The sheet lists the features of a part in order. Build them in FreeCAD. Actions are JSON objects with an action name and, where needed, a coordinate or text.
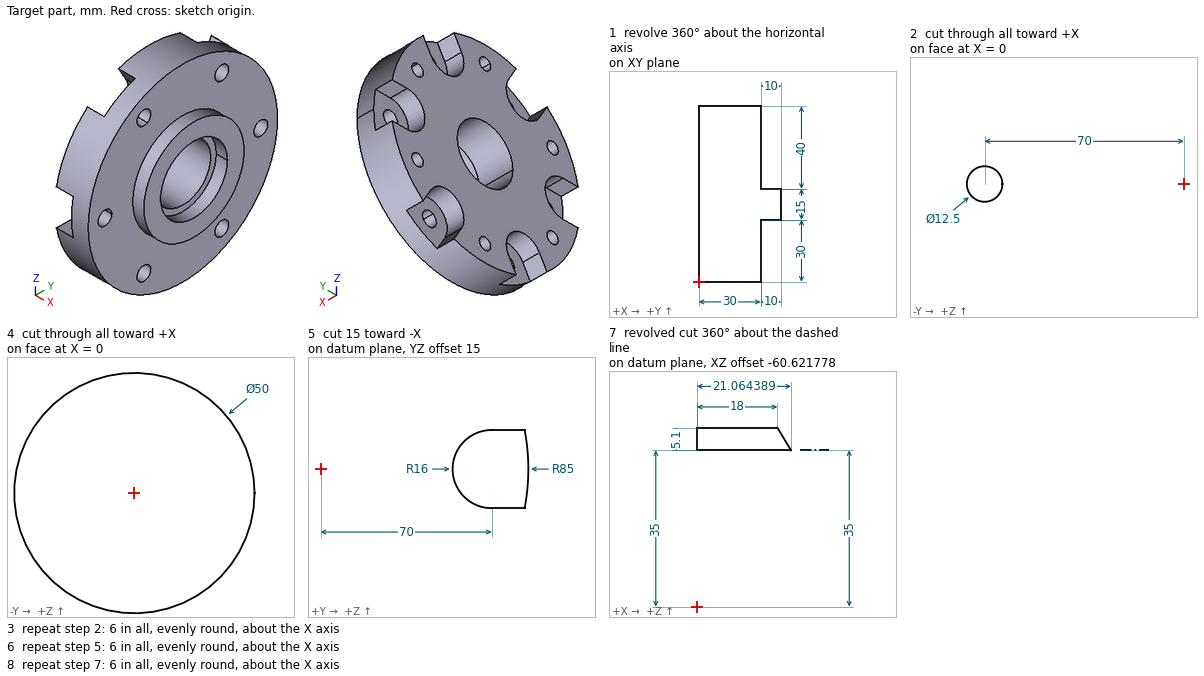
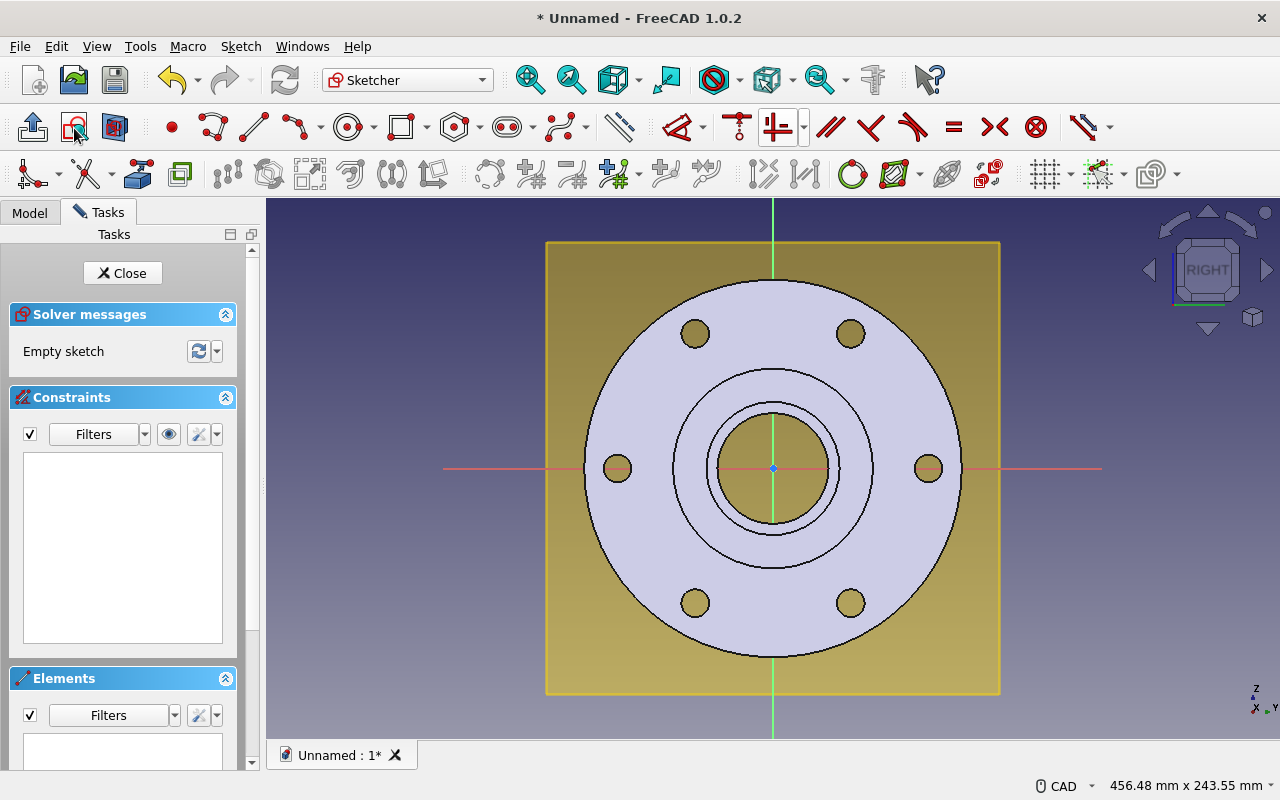
{"action": "left_click", "coordinate": [115, 128]}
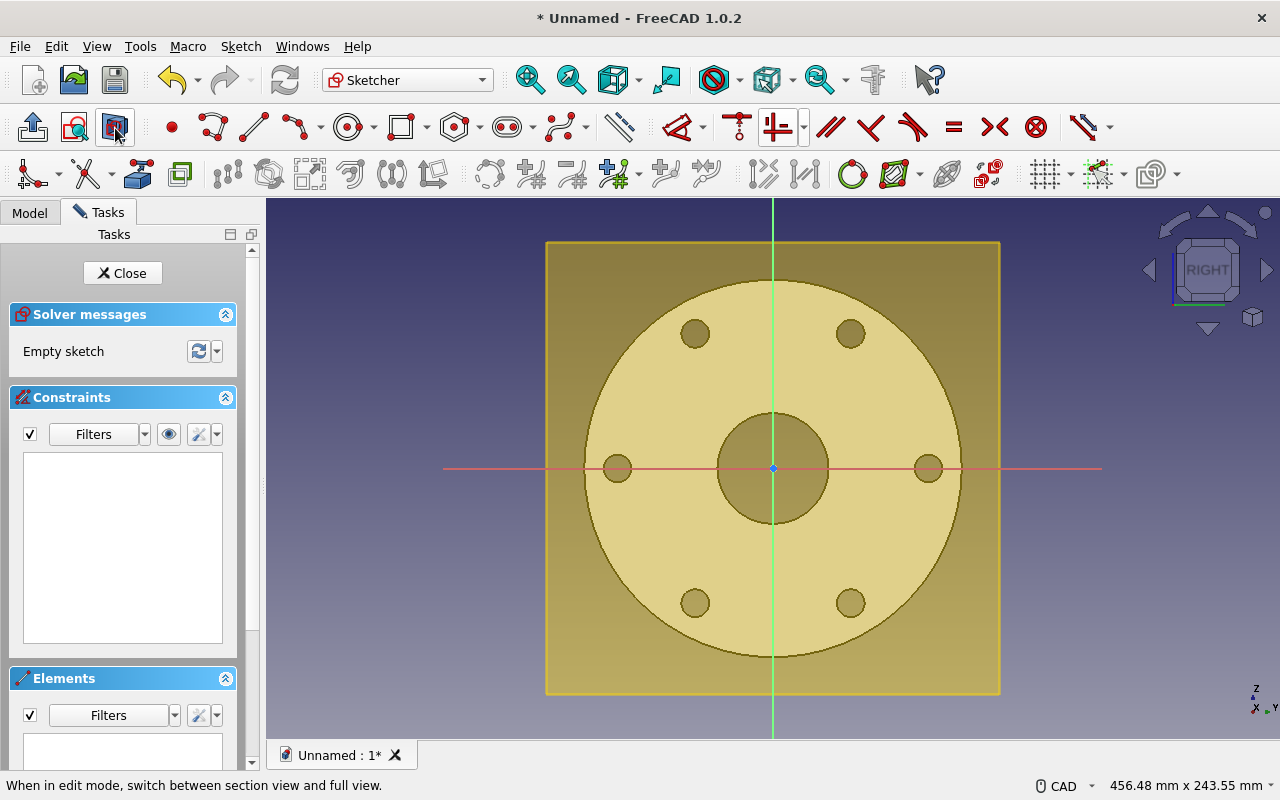
{"action": "scroll", "coordinate": [984, 469], "scroll_direction": "up", "scroll_amount": 8}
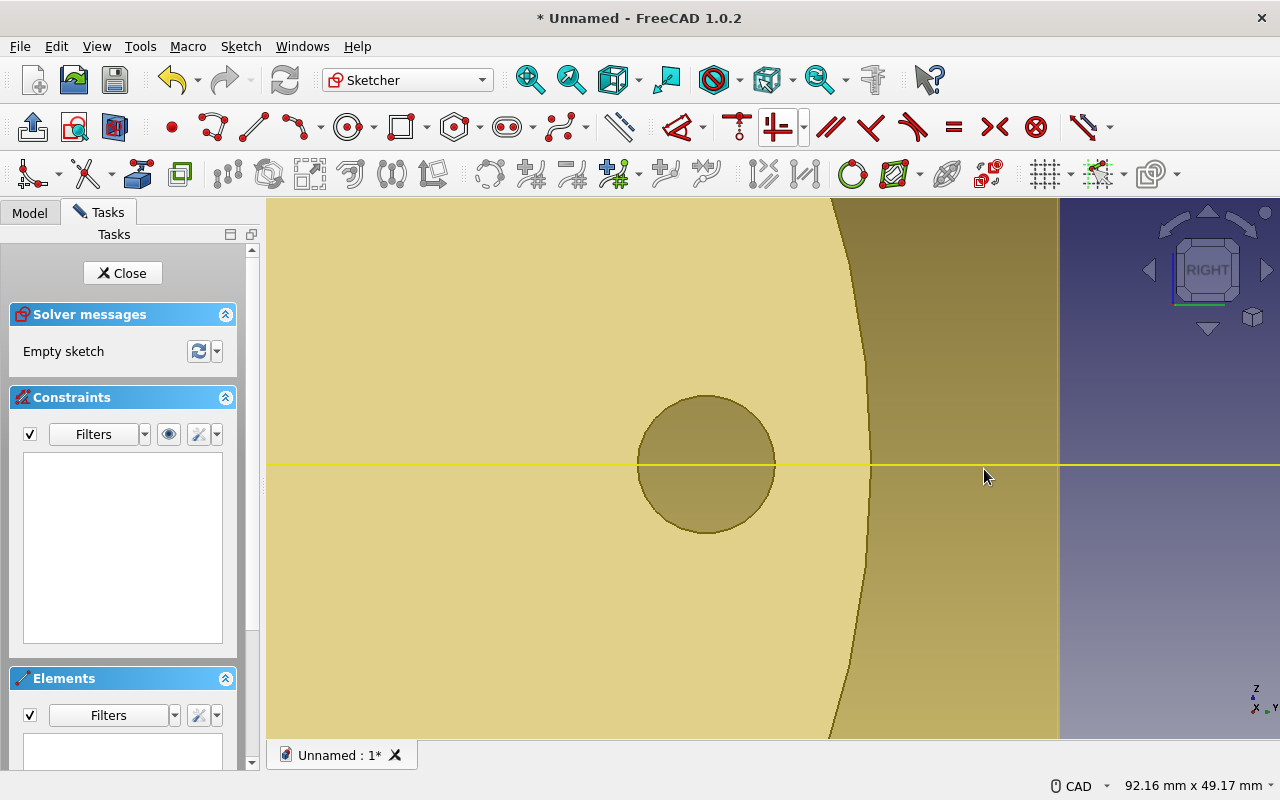
{"action": "left_click", "coordinate": [254, 128]}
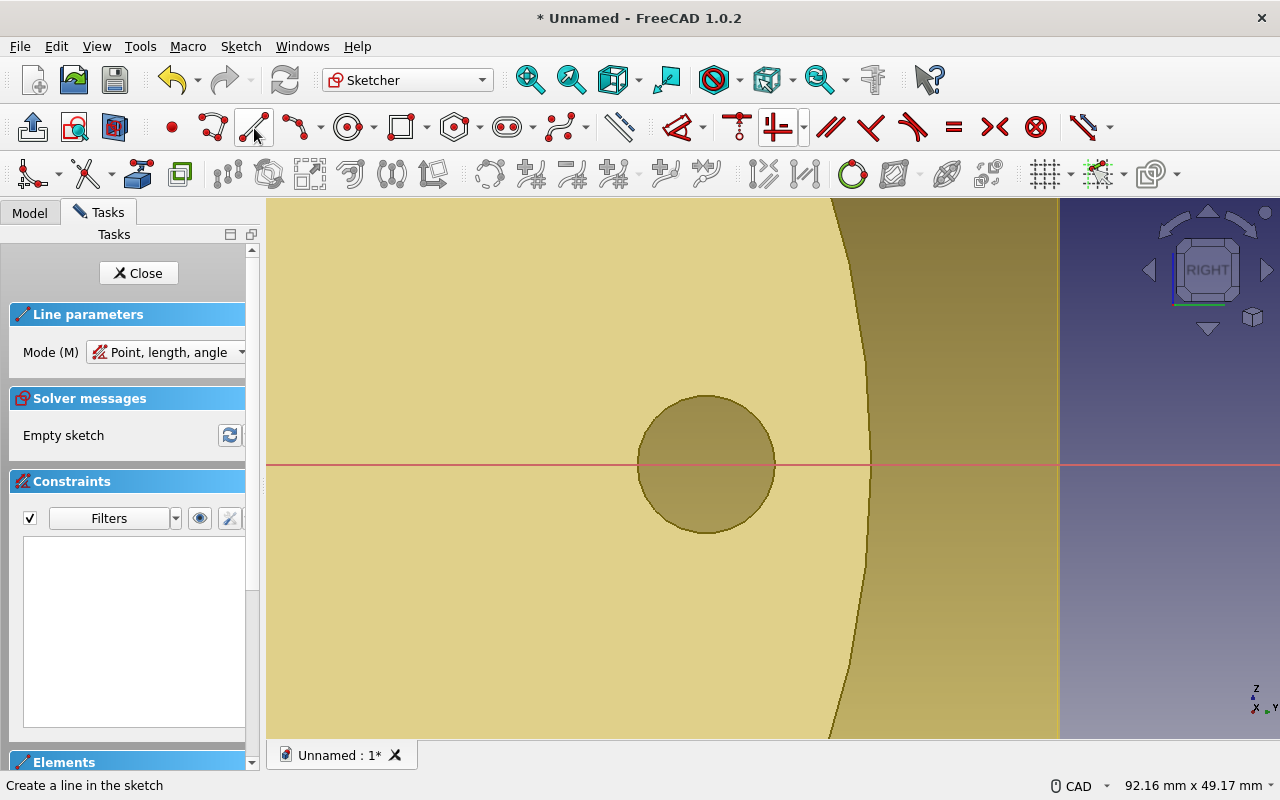
{"action": "left_click", "coordinate": [855, 641]}
{"action": "left_click", "coordinate": [706, 641]}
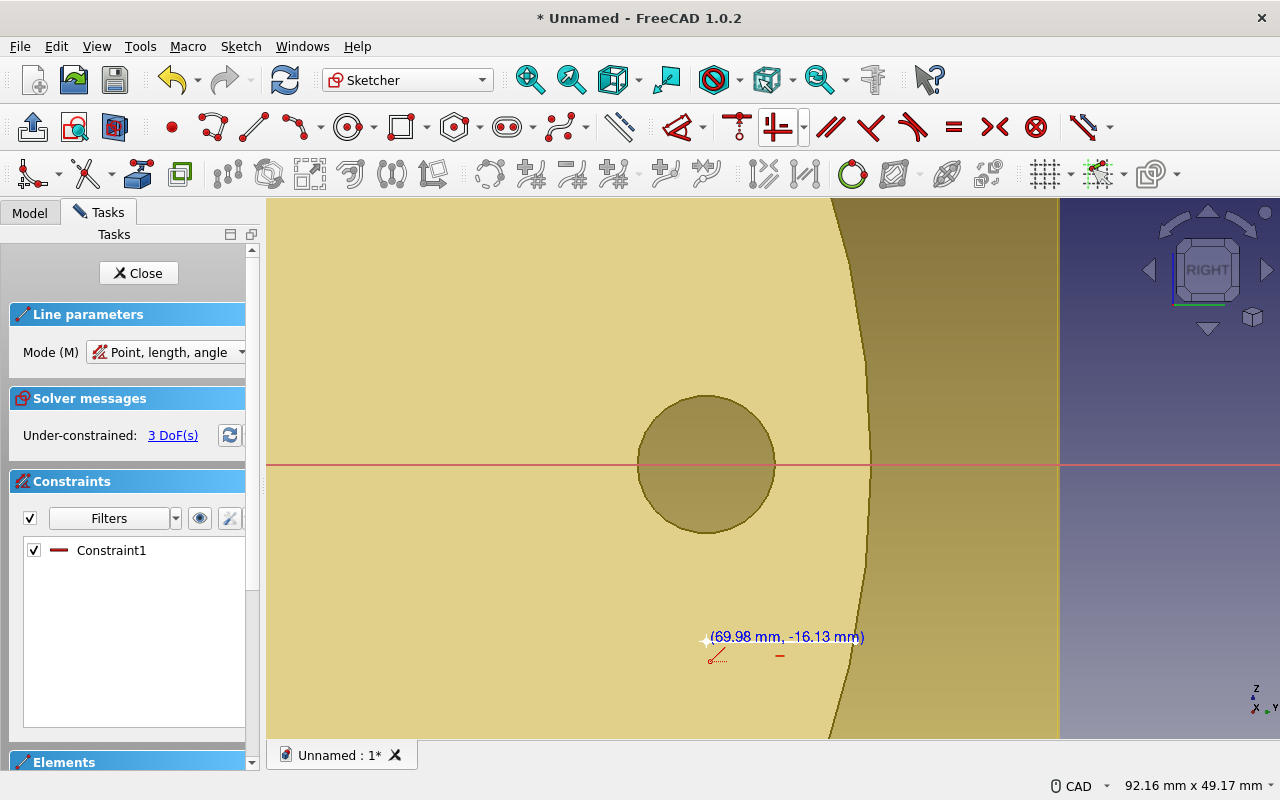
{"action": "left_click", "coordinate": [706, 289]}
{"action": "left_click", "coordinate": [855, 289]}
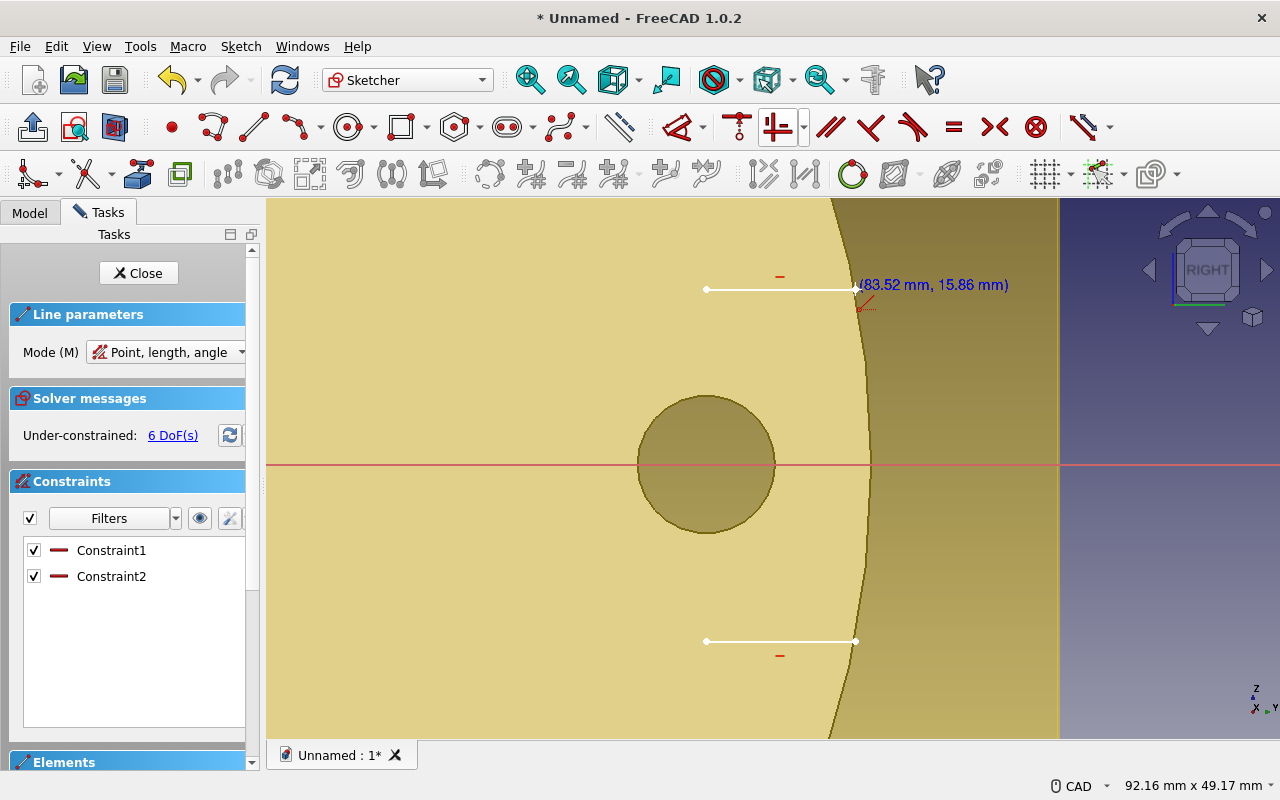
{"action": "left_click", "coordinate": [294, 128]}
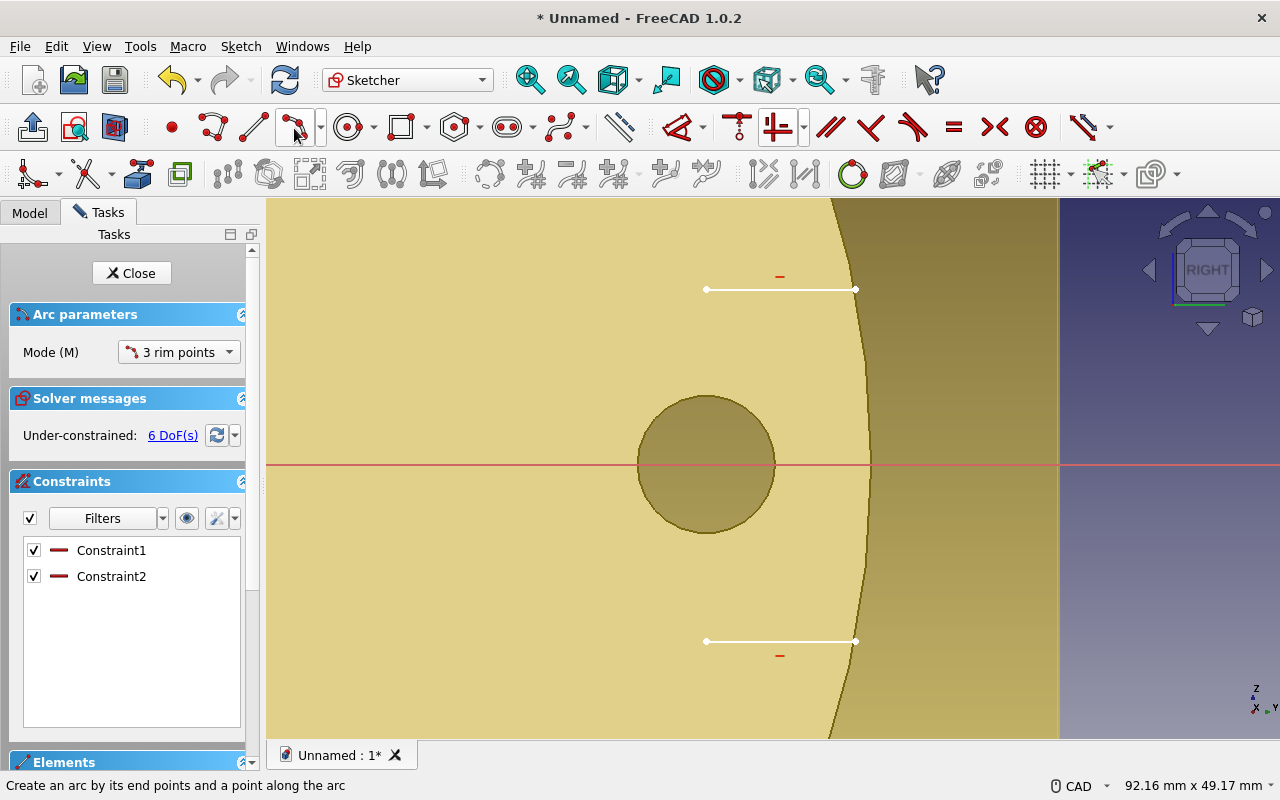
{"action": "left_click", "coordinate": [706, 642]}
{"action": "left_click", "coordinate": [706, 290]}
{"action": "left_click", "coordinate": [539, 410]}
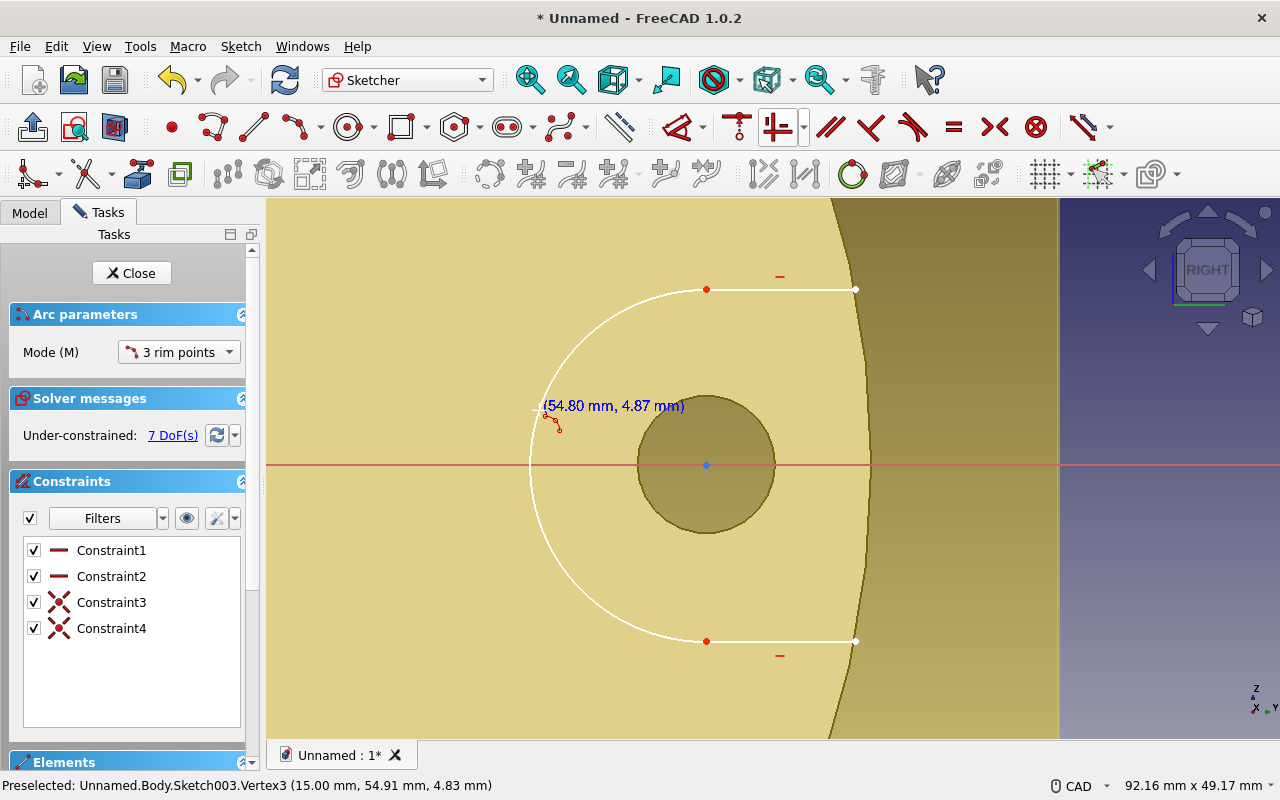
{"action": "left_click", "coordinate": [855, 290]}
{"action": "left_click", "coordinate": [855, 642]}
{"action": "left_click", "coordinate": [871, 500]}
{"action": "key", "text": "Escape"}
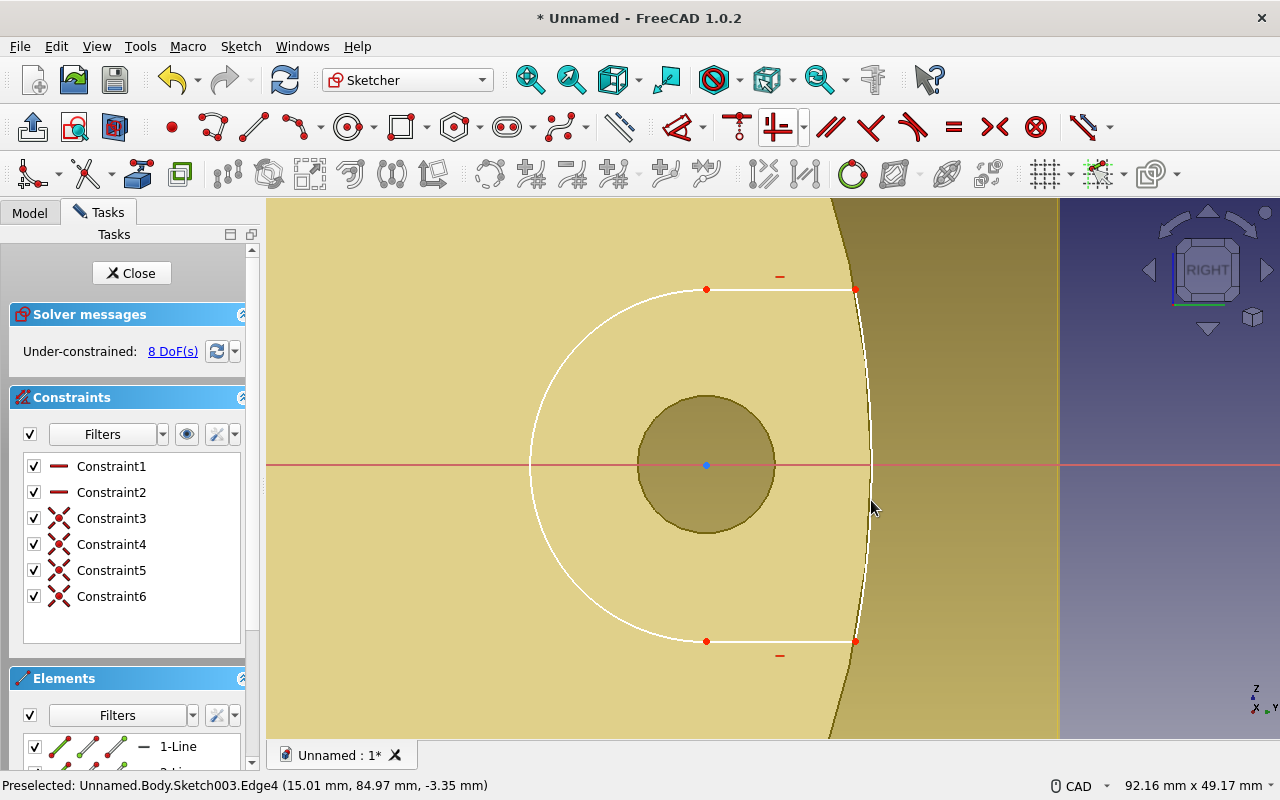
{"action": "left_click", "coordinate": [810, 642]}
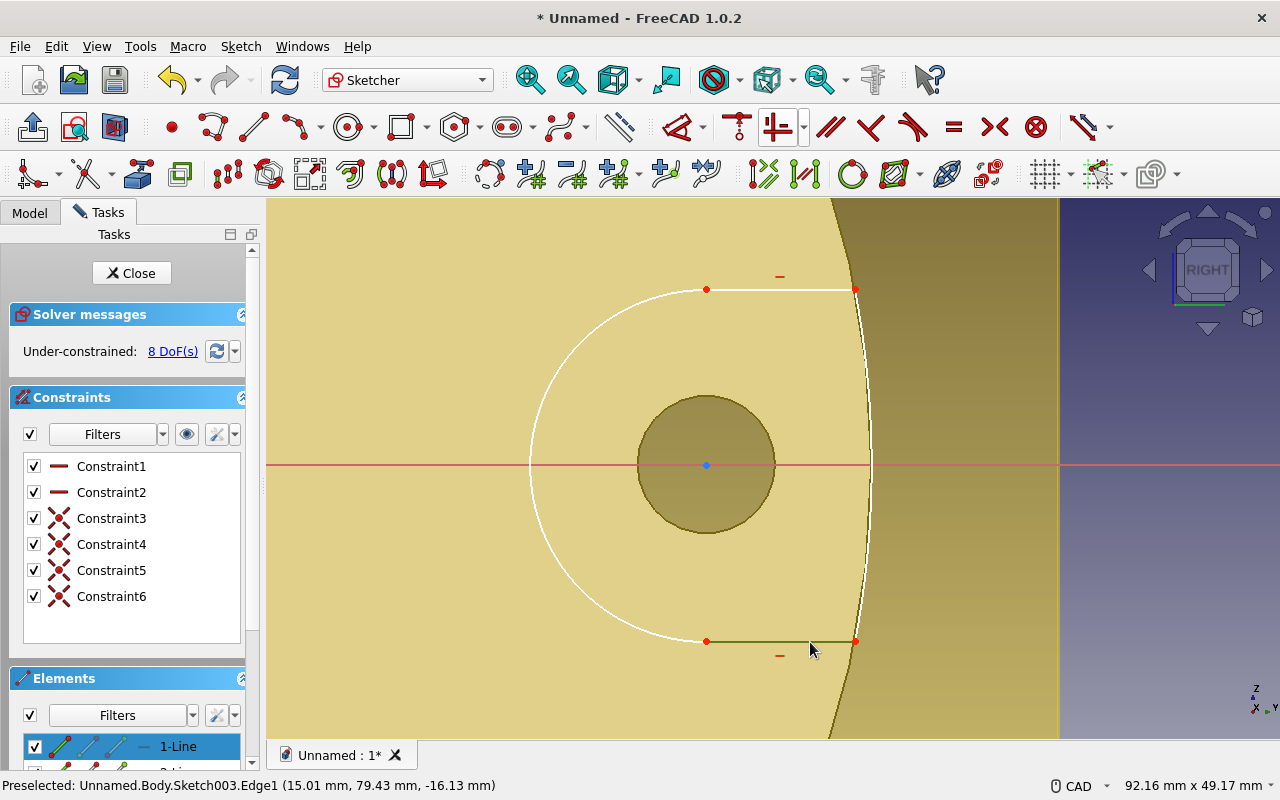
{"action": "left_click", "coordinate": [564, 363]}